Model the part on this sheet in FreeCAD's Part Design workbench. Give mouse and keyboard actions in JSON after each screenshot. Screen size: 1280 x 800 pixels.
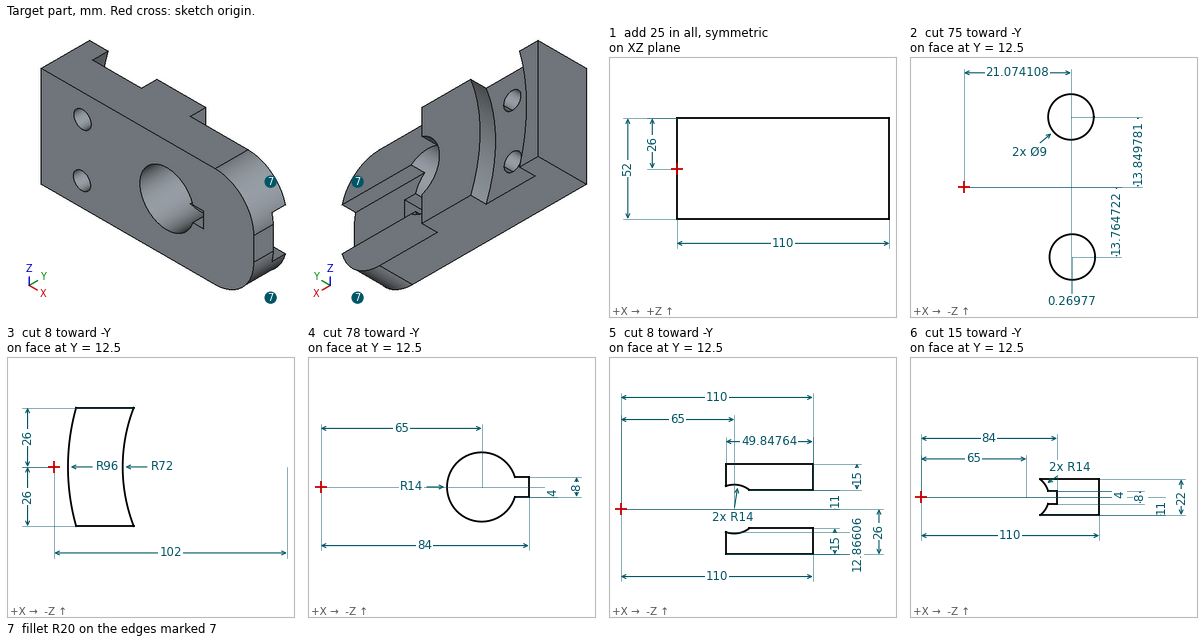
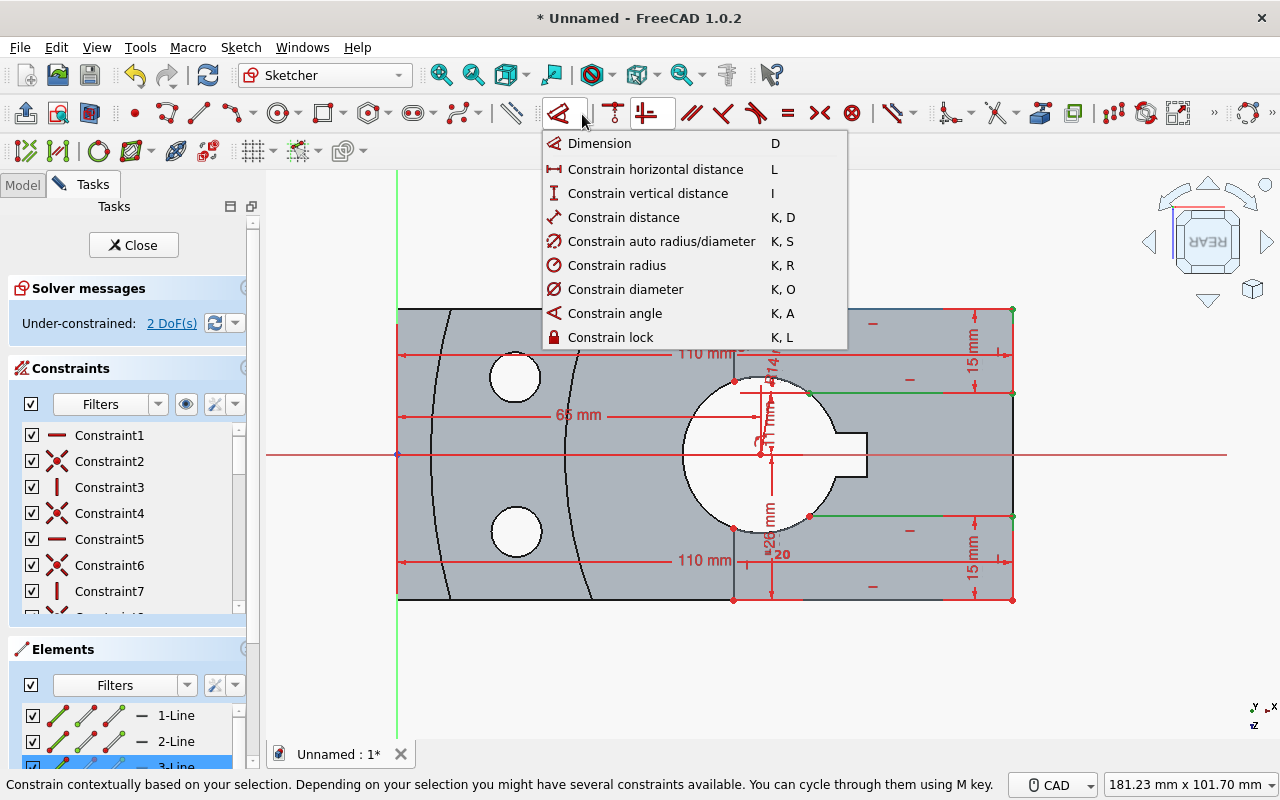
{"action": "left_click", "coordinate": [695, 169]}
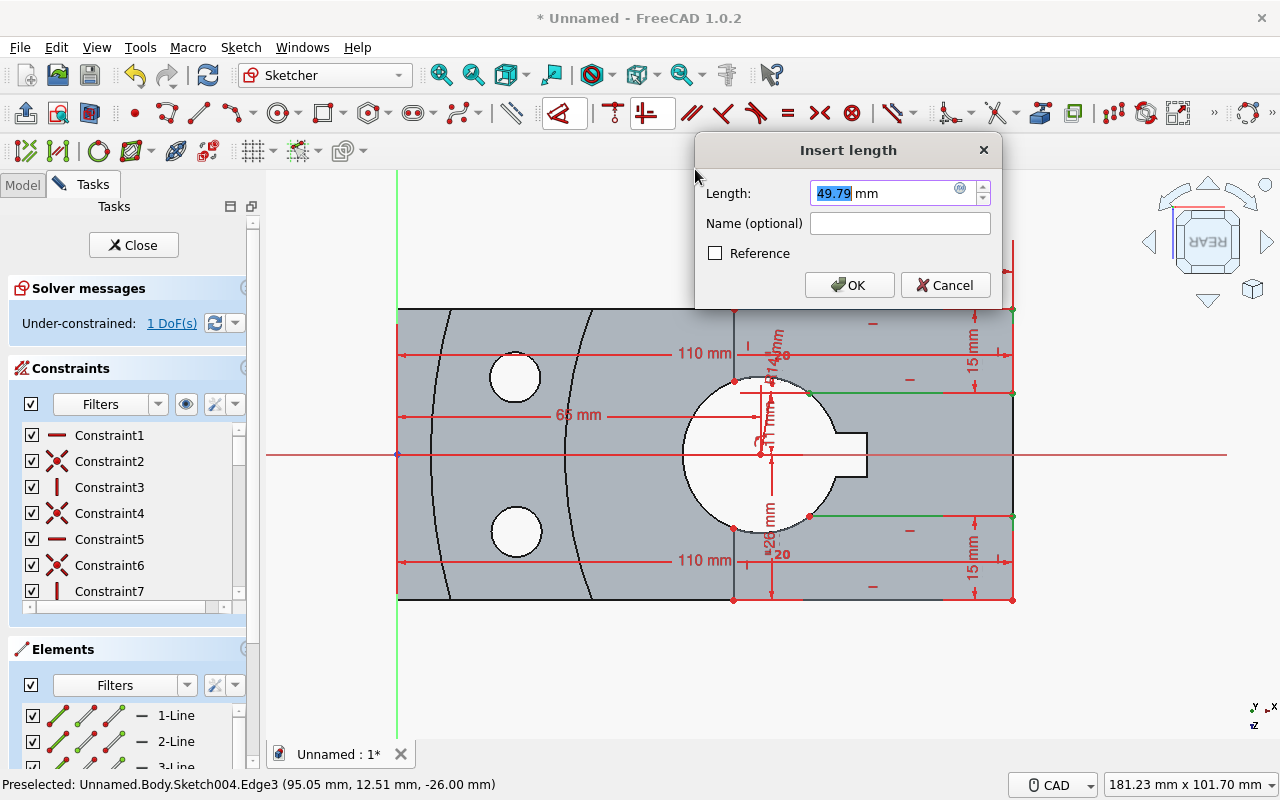
{"action": "type", "text": "49.84764"}
{"action": "key", "text": "Return"}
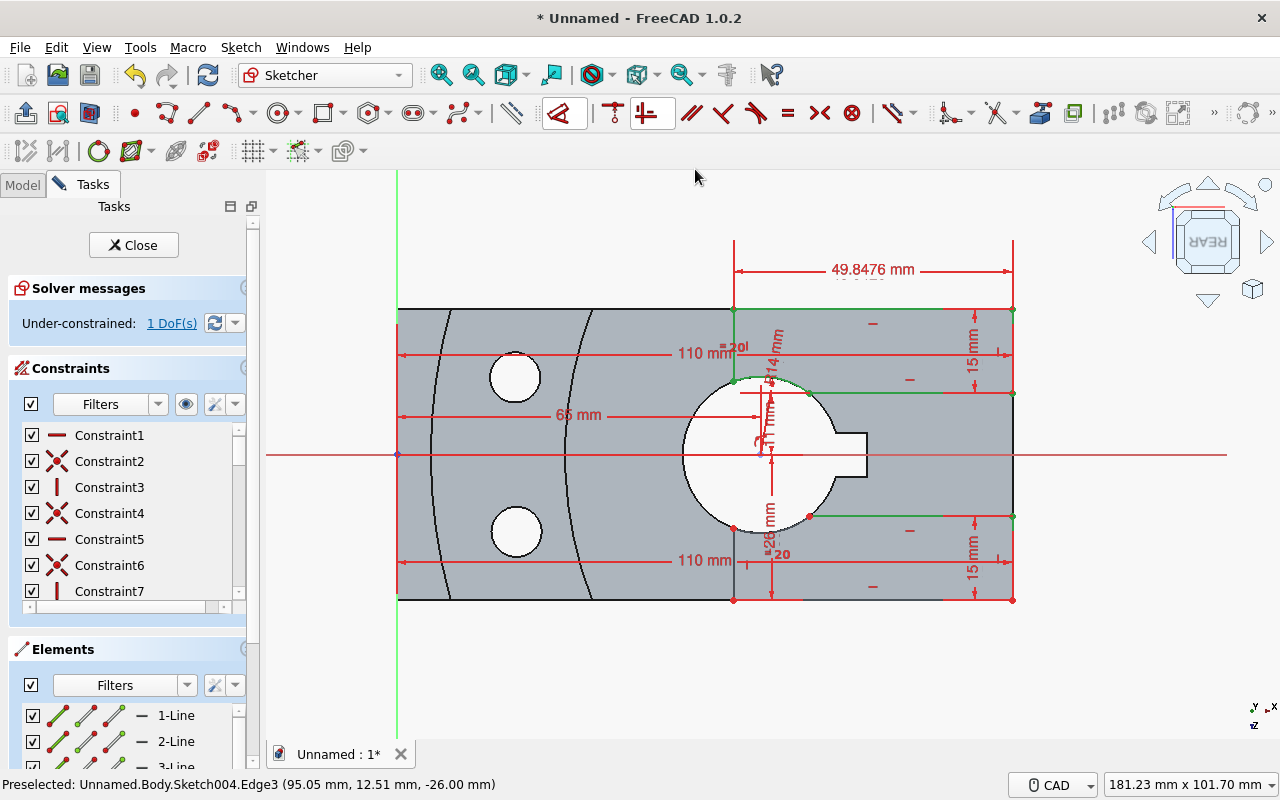
{"action": "left_click", "coordinate": [734, 550]}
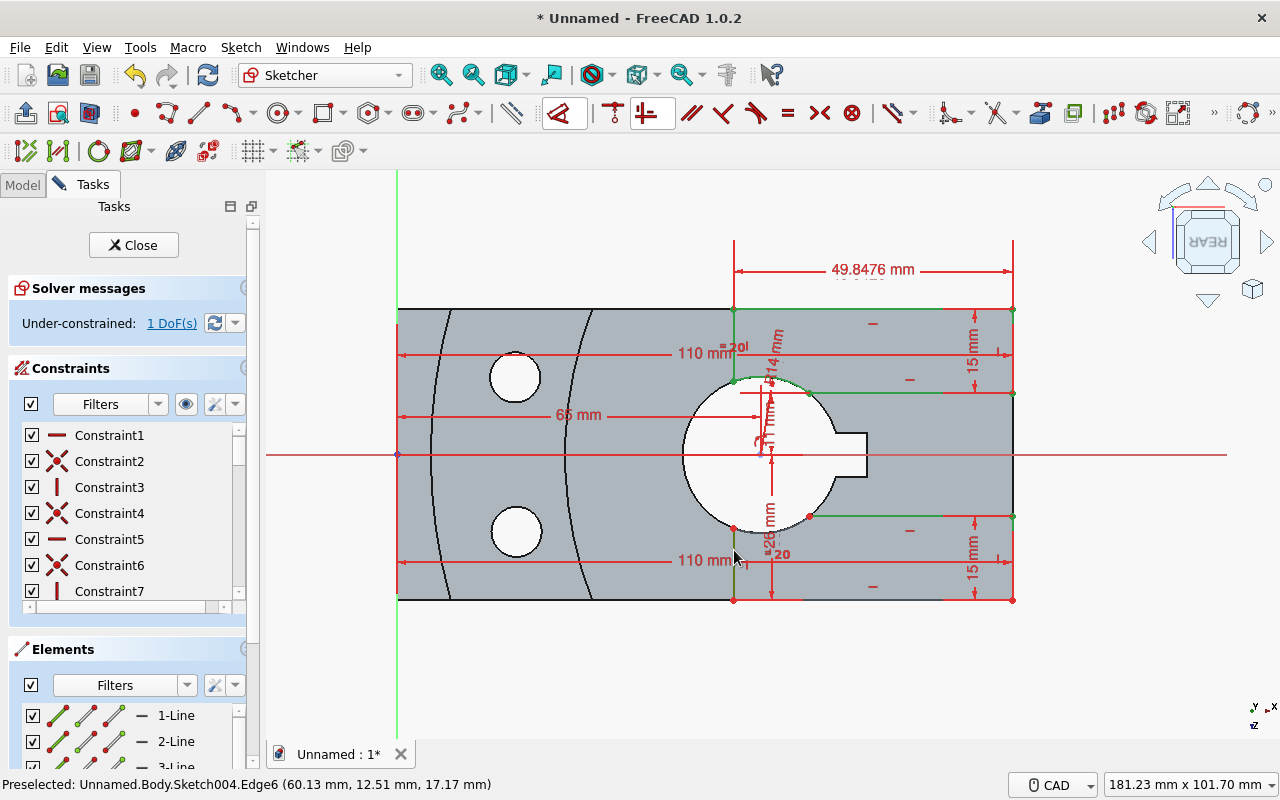
{"action": "left_click", "coordinate": [582, 114]}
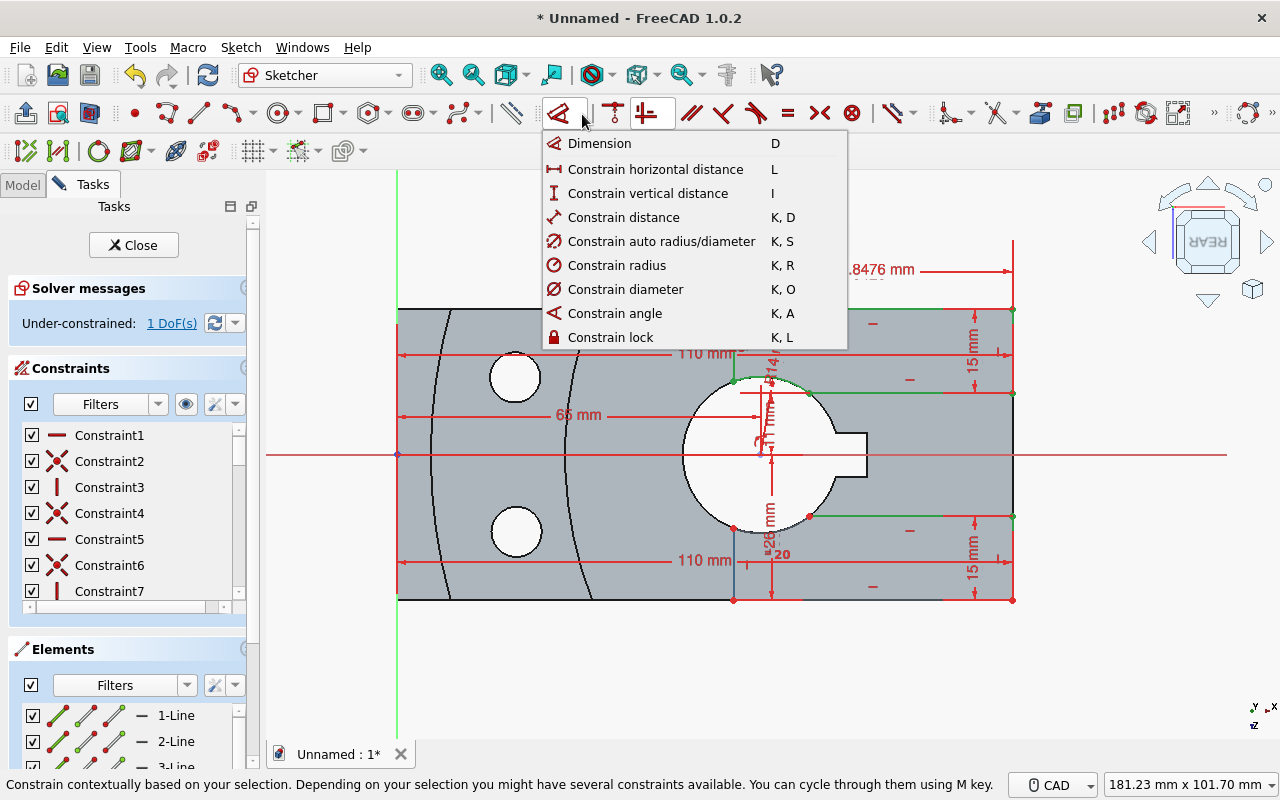
{"action": "left_click", "coordinate": [695, 193]}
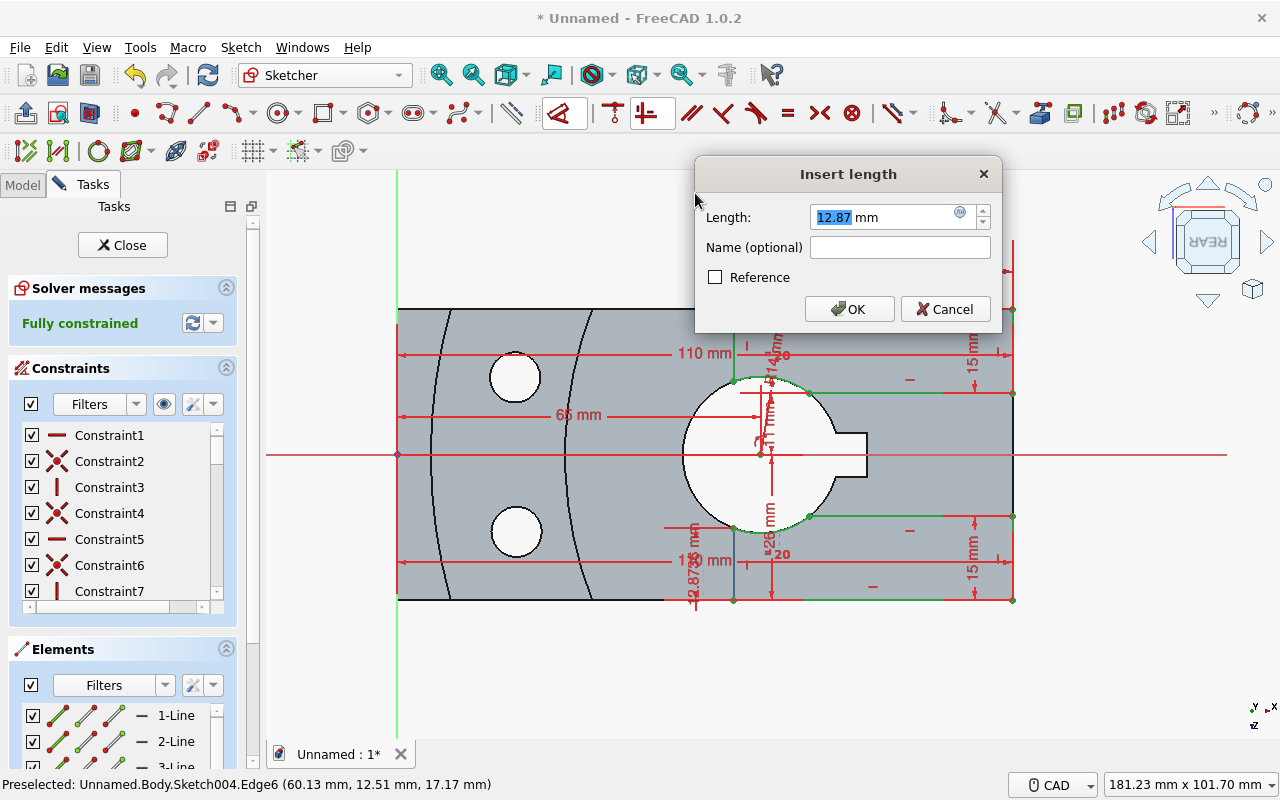
{"action": "type", "text": "12.86606"}
{"action": "key", "text": "Return"}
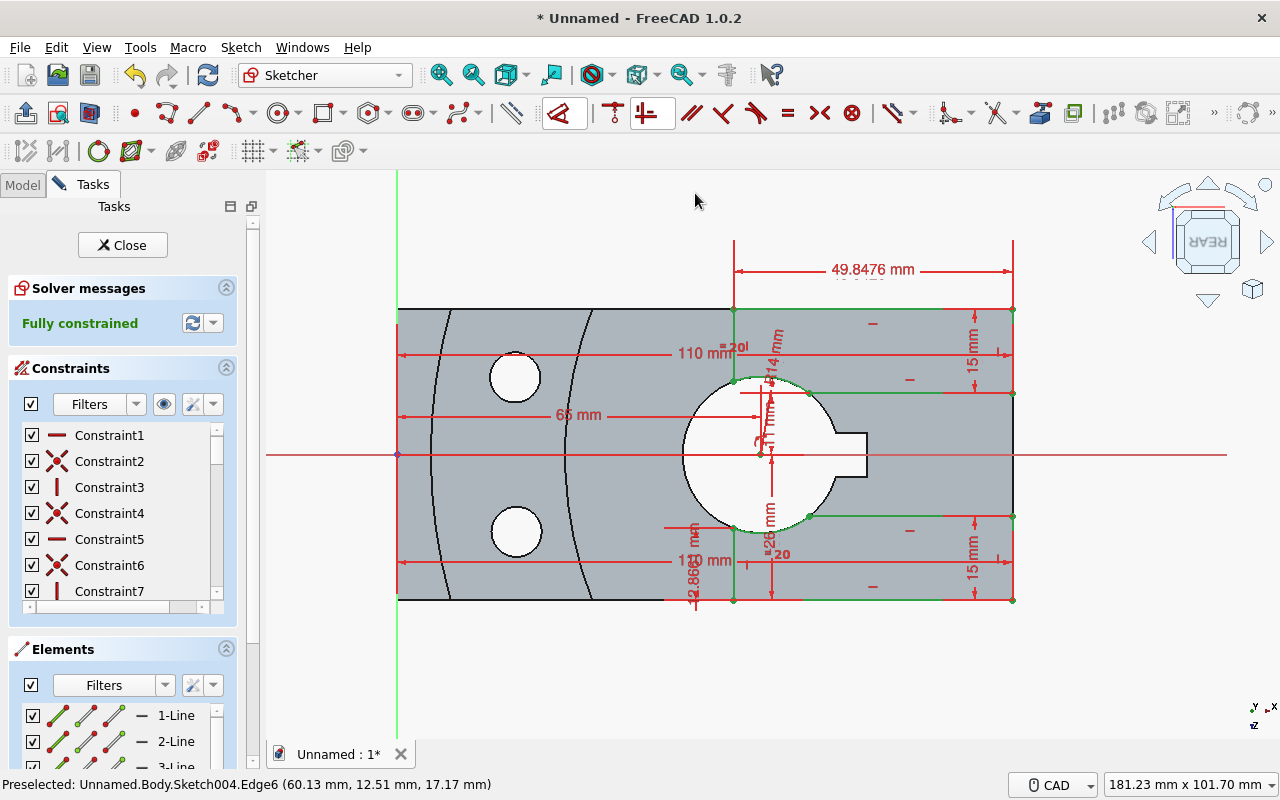
{"action": "left_click", "coordinate": [123, 245]}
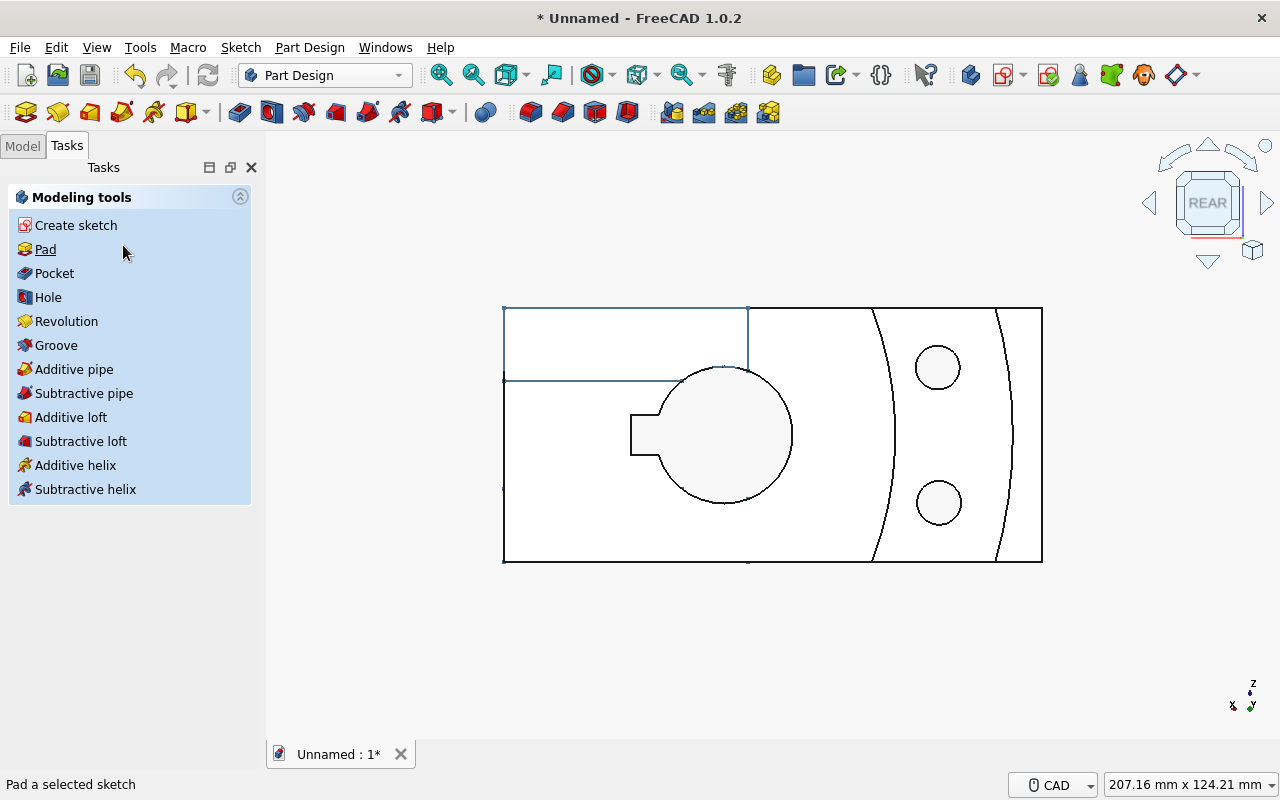
{"action": "left_click", "coordinate": [240, 112]}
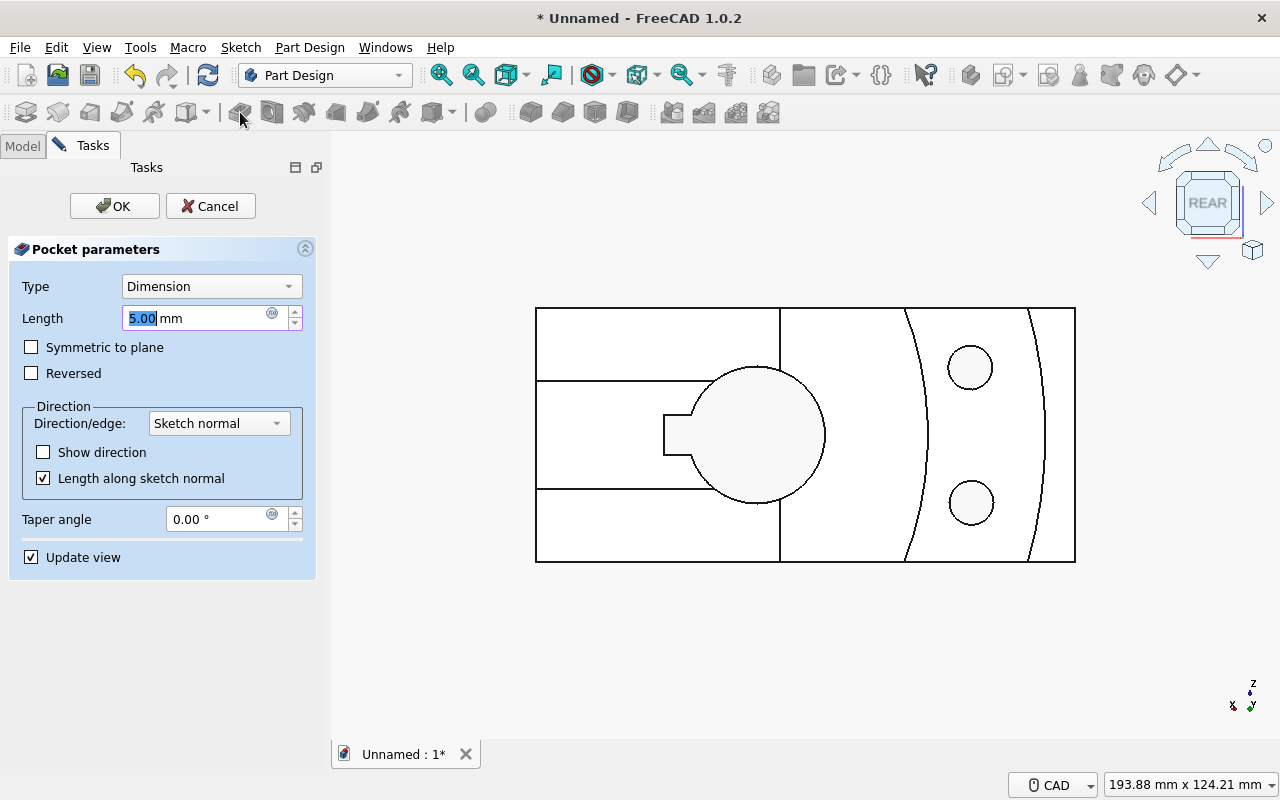
{"action": "type", "text": "8"}
{"action": "key", "text": "Tab"}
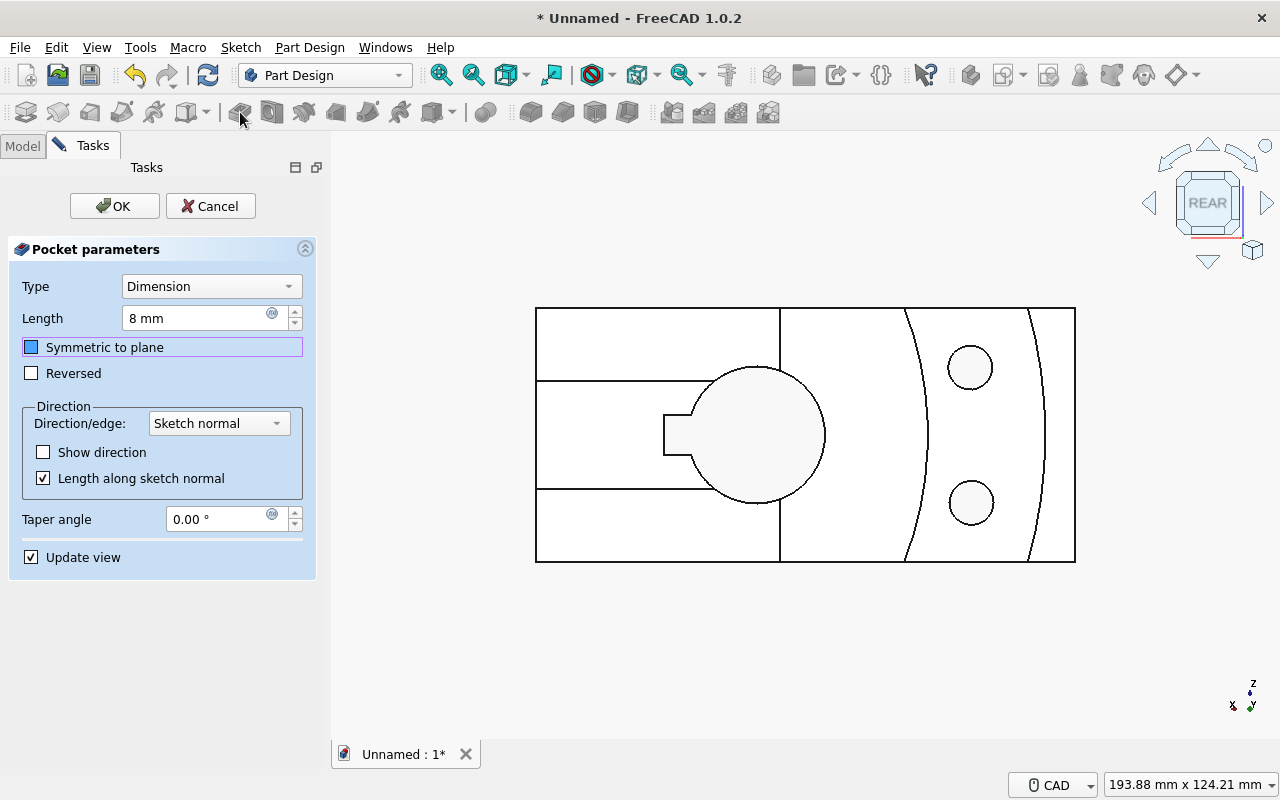
{"action": "left_click", "coordinate": [115, 206]}